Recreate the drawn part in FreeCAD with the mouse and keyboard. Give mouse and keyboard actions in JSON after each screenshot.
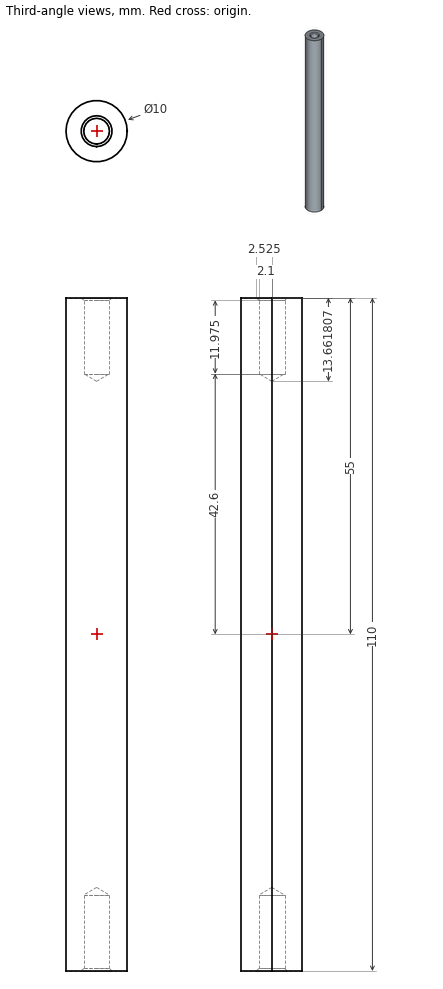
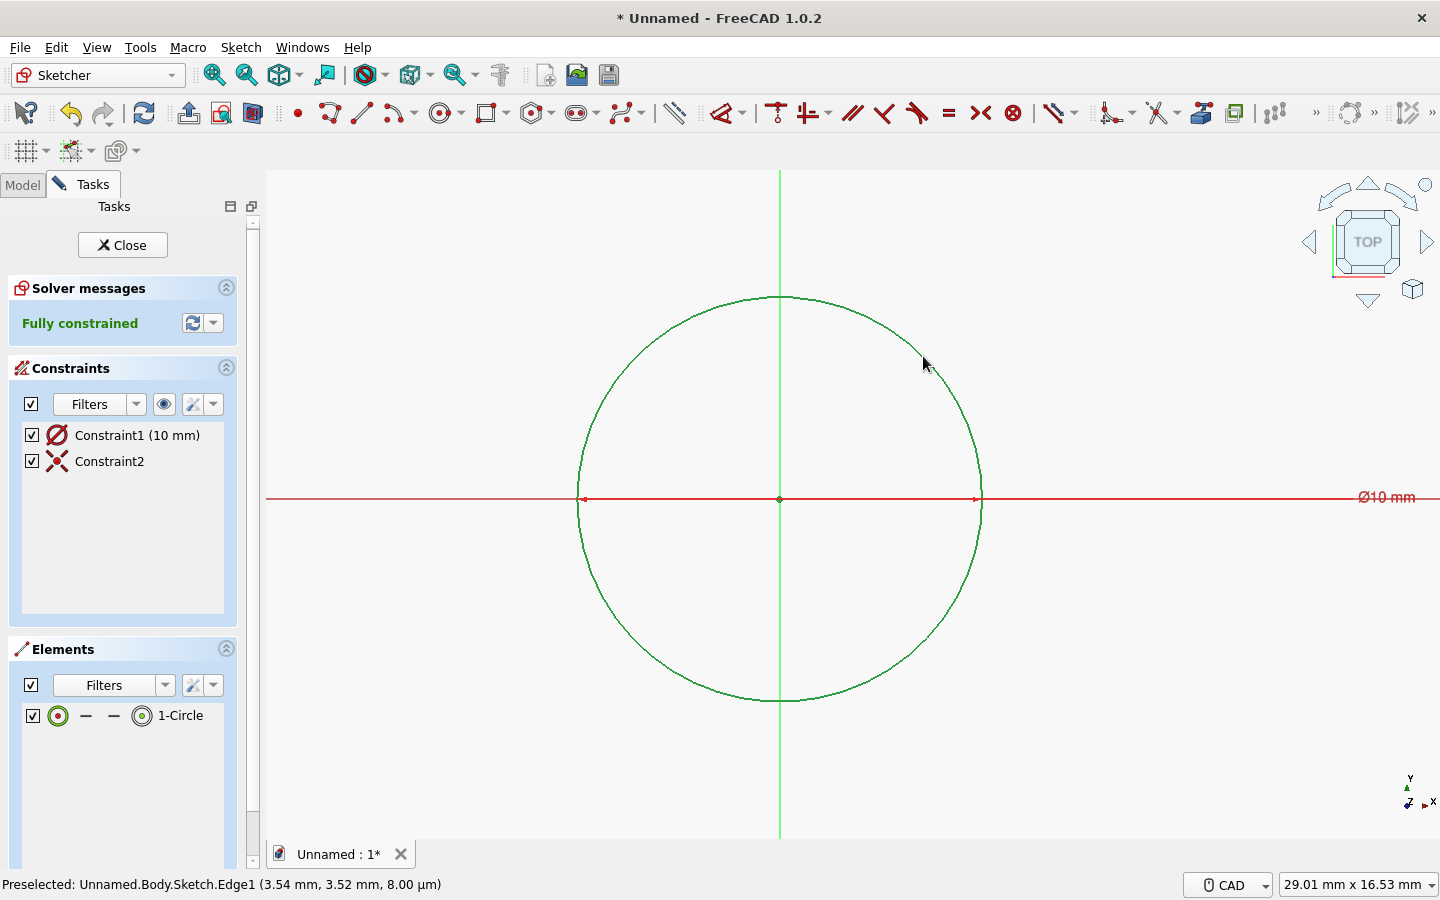
{"action": "left_click", "coordinate": [123, 245]}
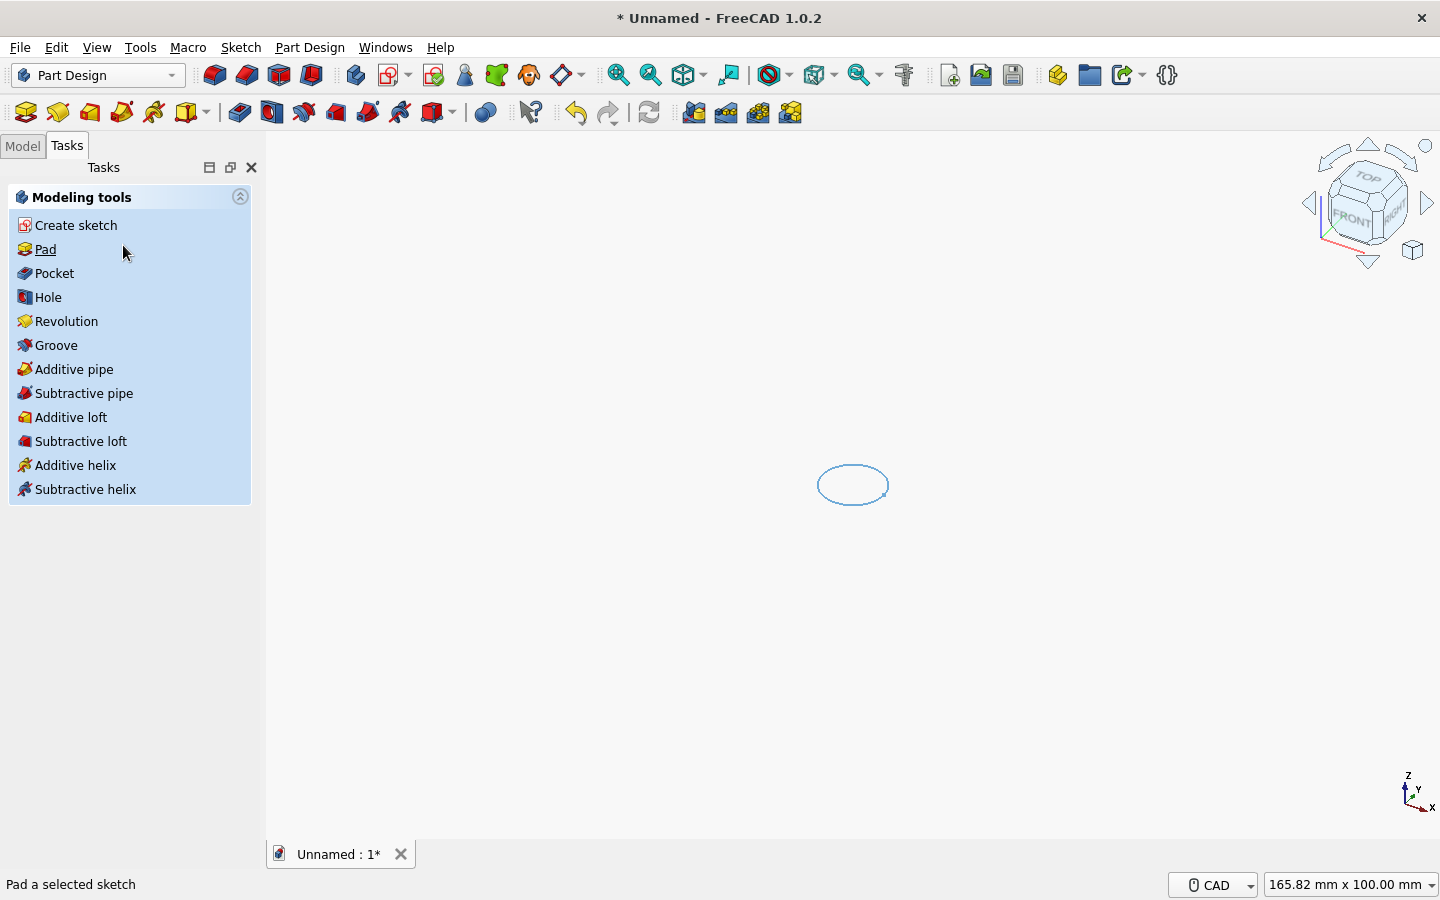
{"action": "left_click", "coordinate": [26, 112]}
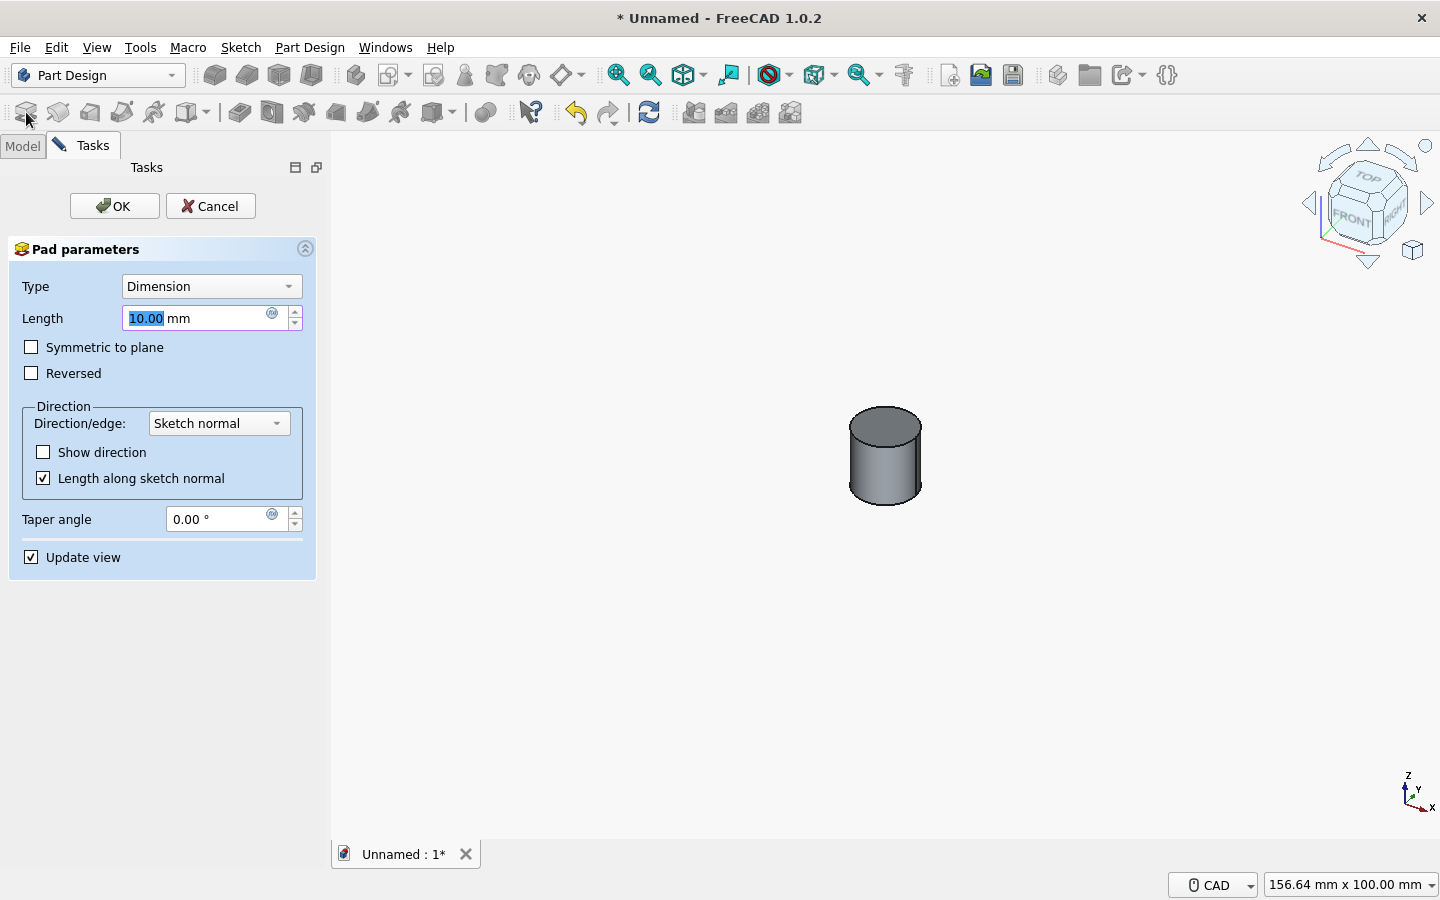
{"action": "type", "text": "110"}
{"action": "key", "text": "Tab"}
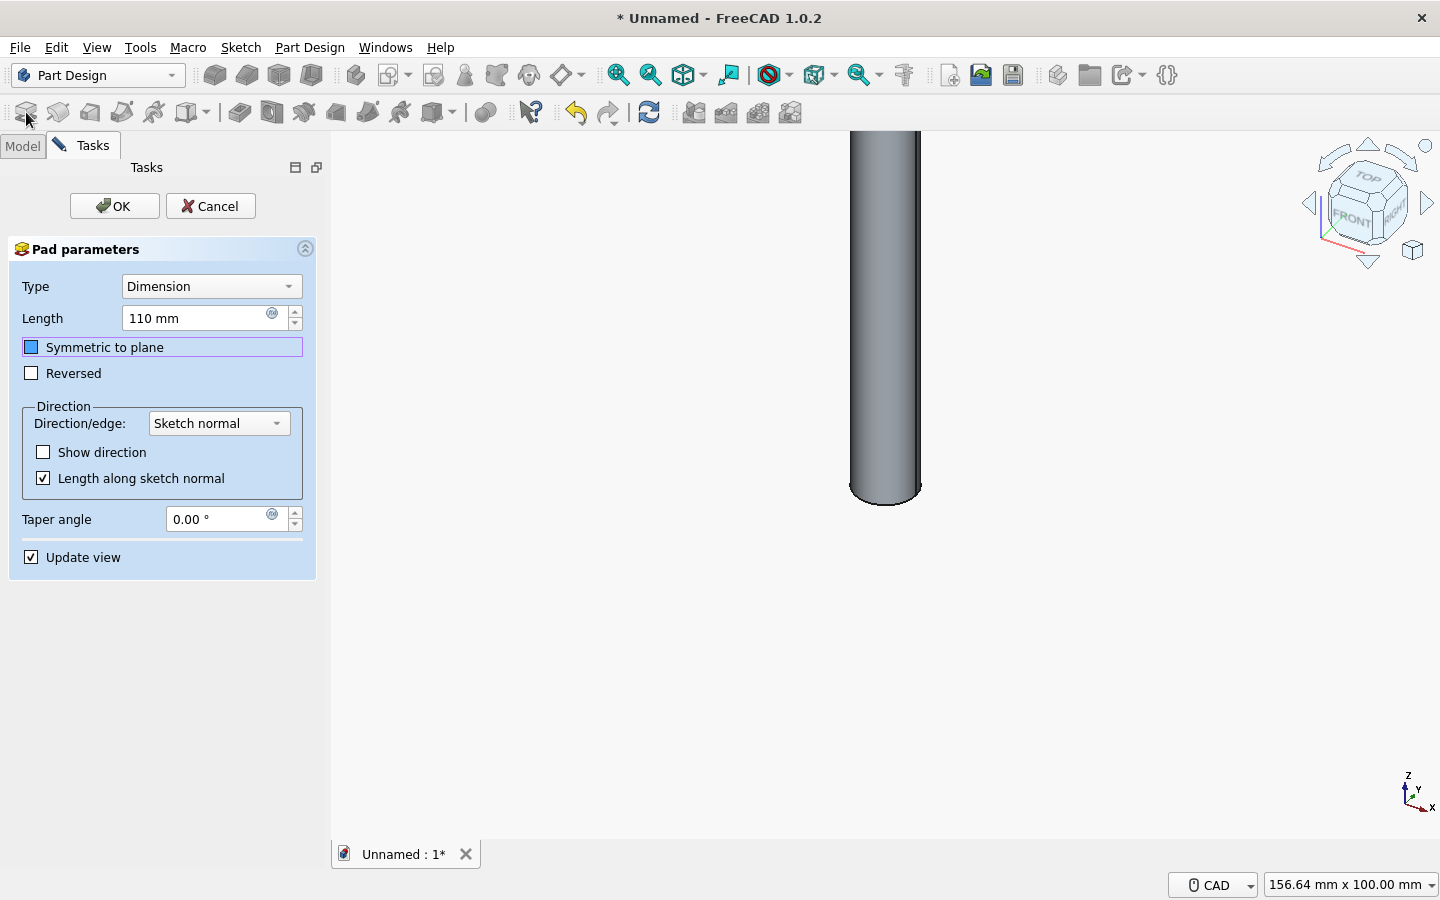
{"action": "left_click", "coordinate": [30, 347]}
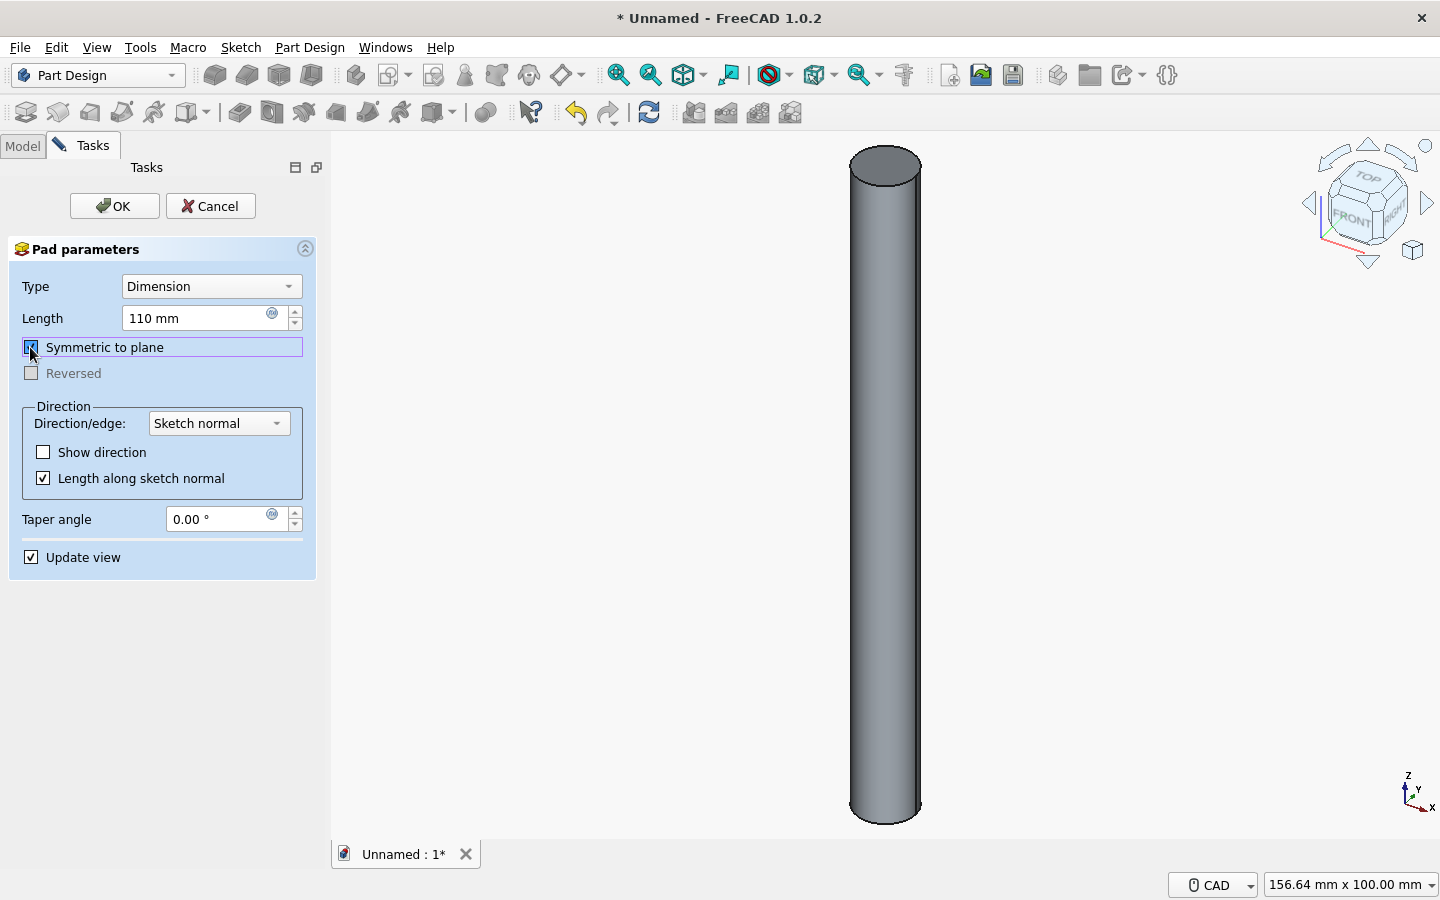
{"action": "left_click", "coordinate": [115, 206]}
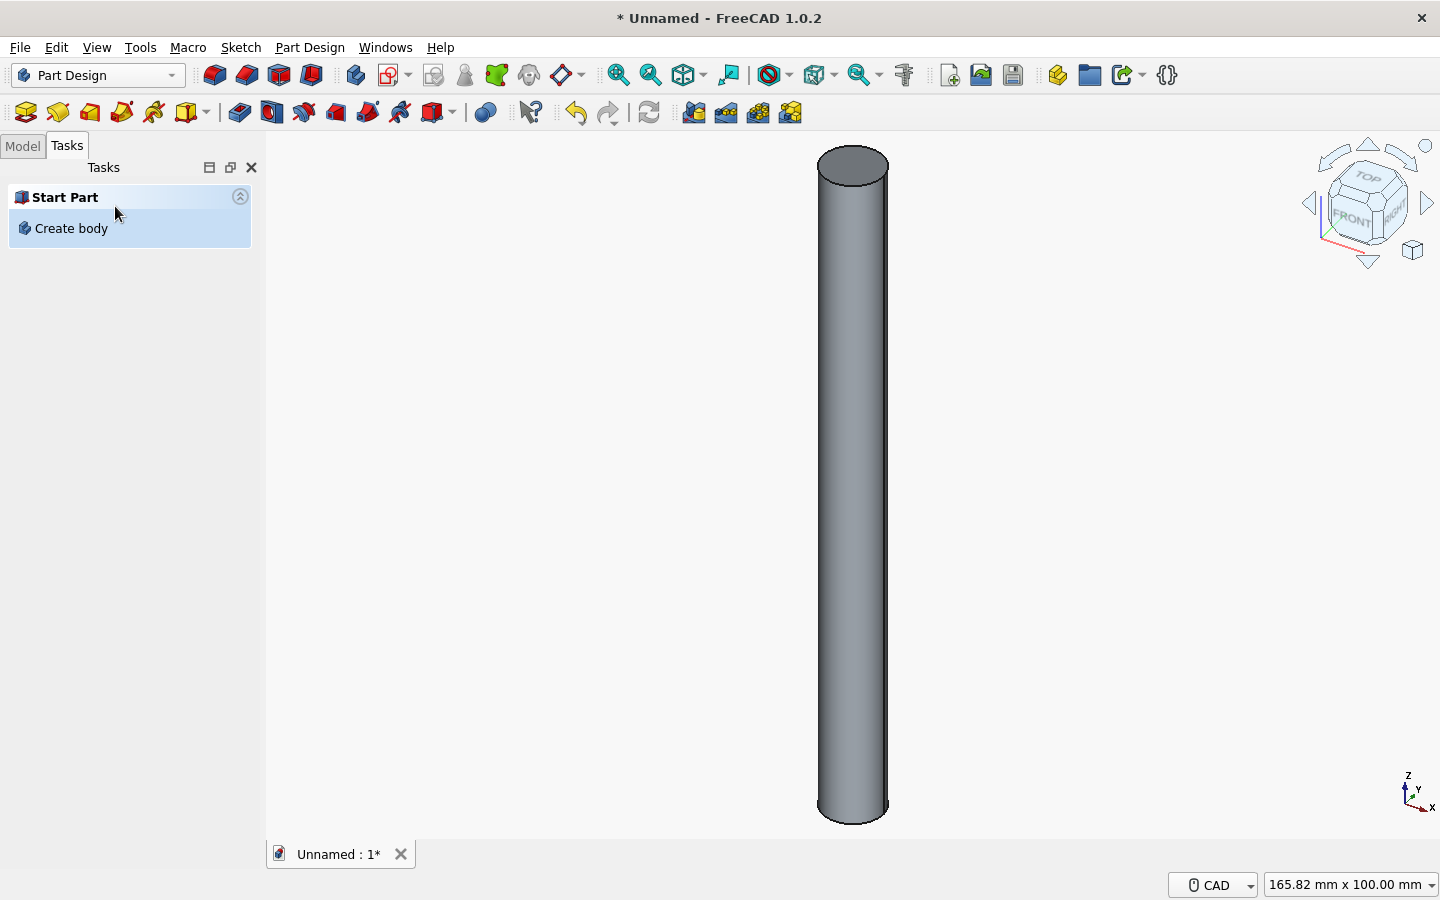
{"action": "left_click", "coordinate": [388, 76]}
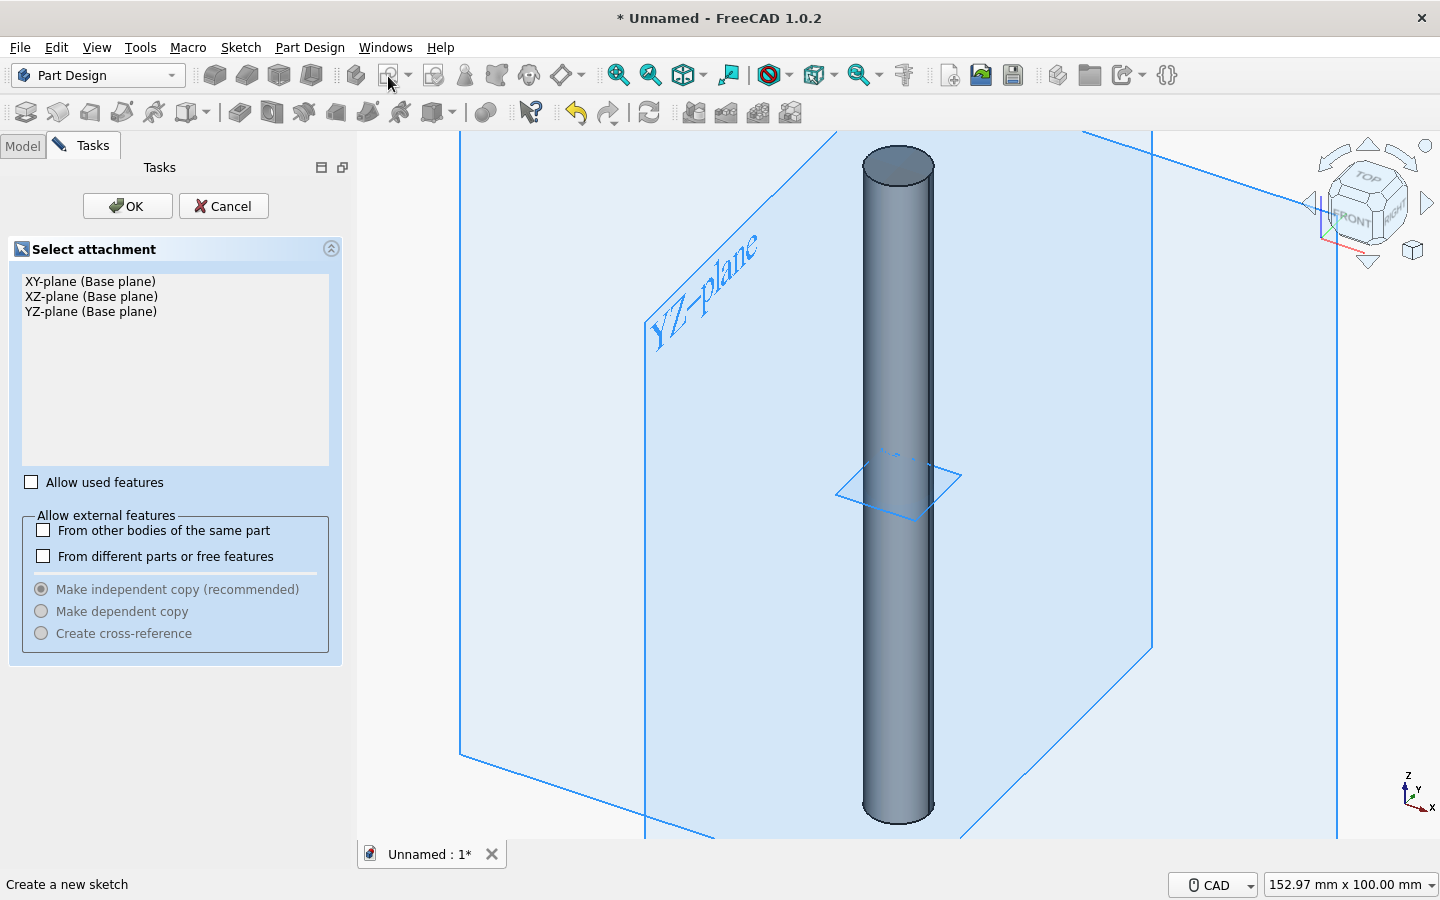
{"action": "left_click", "coordinate": [82, 312]}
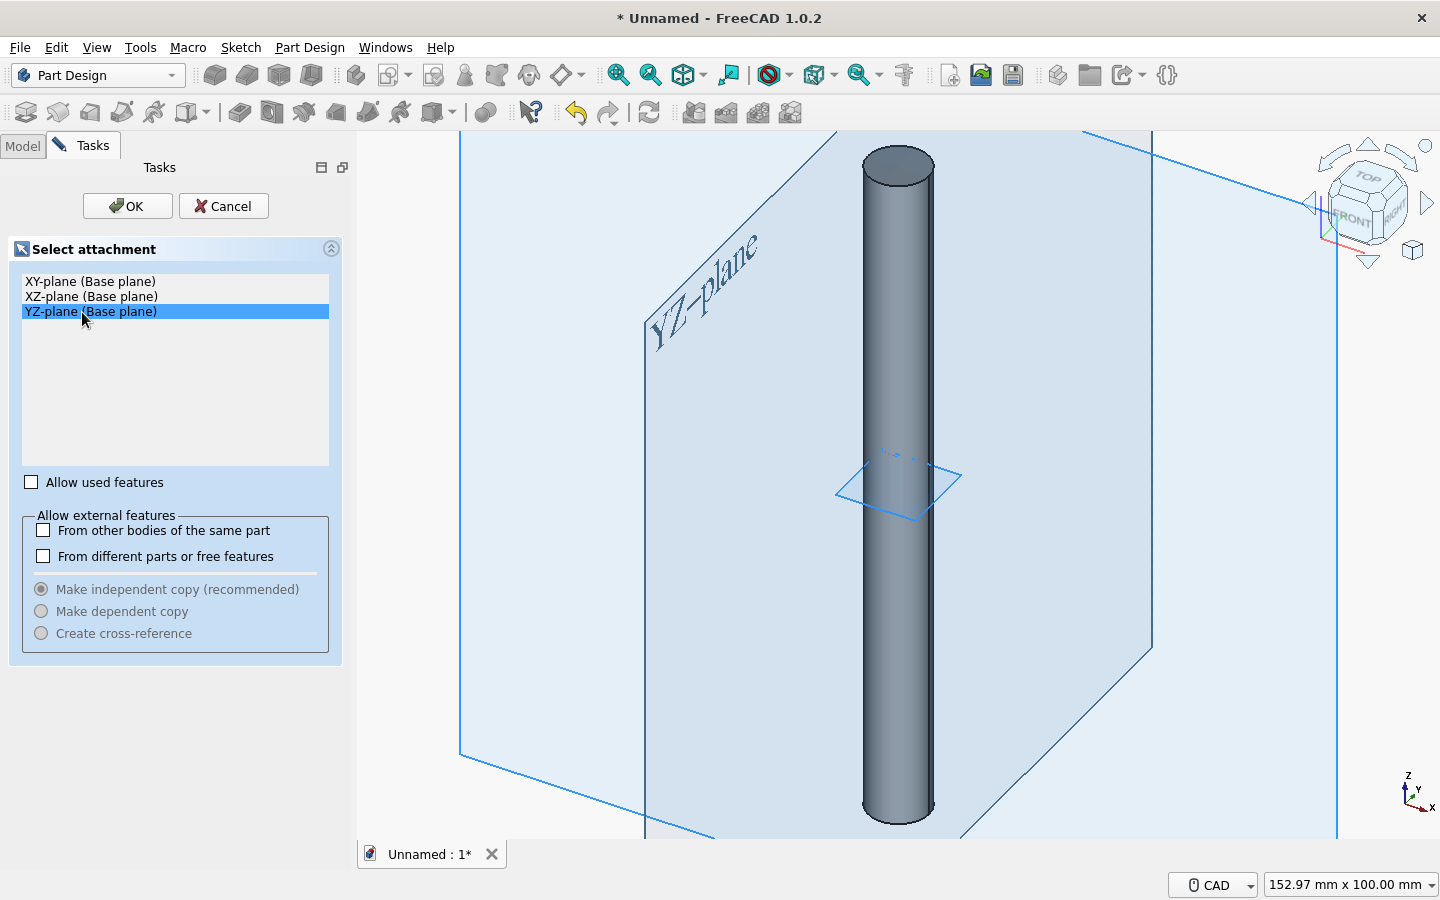
{"action": "left_click", "coordinate": [128, 206]}